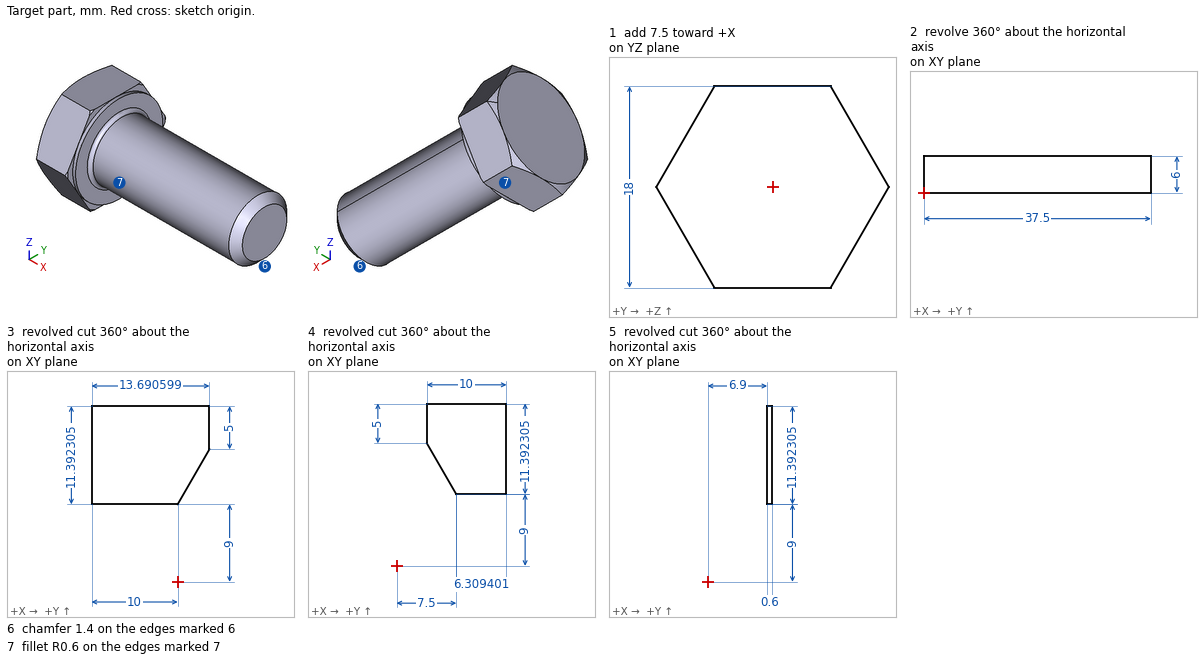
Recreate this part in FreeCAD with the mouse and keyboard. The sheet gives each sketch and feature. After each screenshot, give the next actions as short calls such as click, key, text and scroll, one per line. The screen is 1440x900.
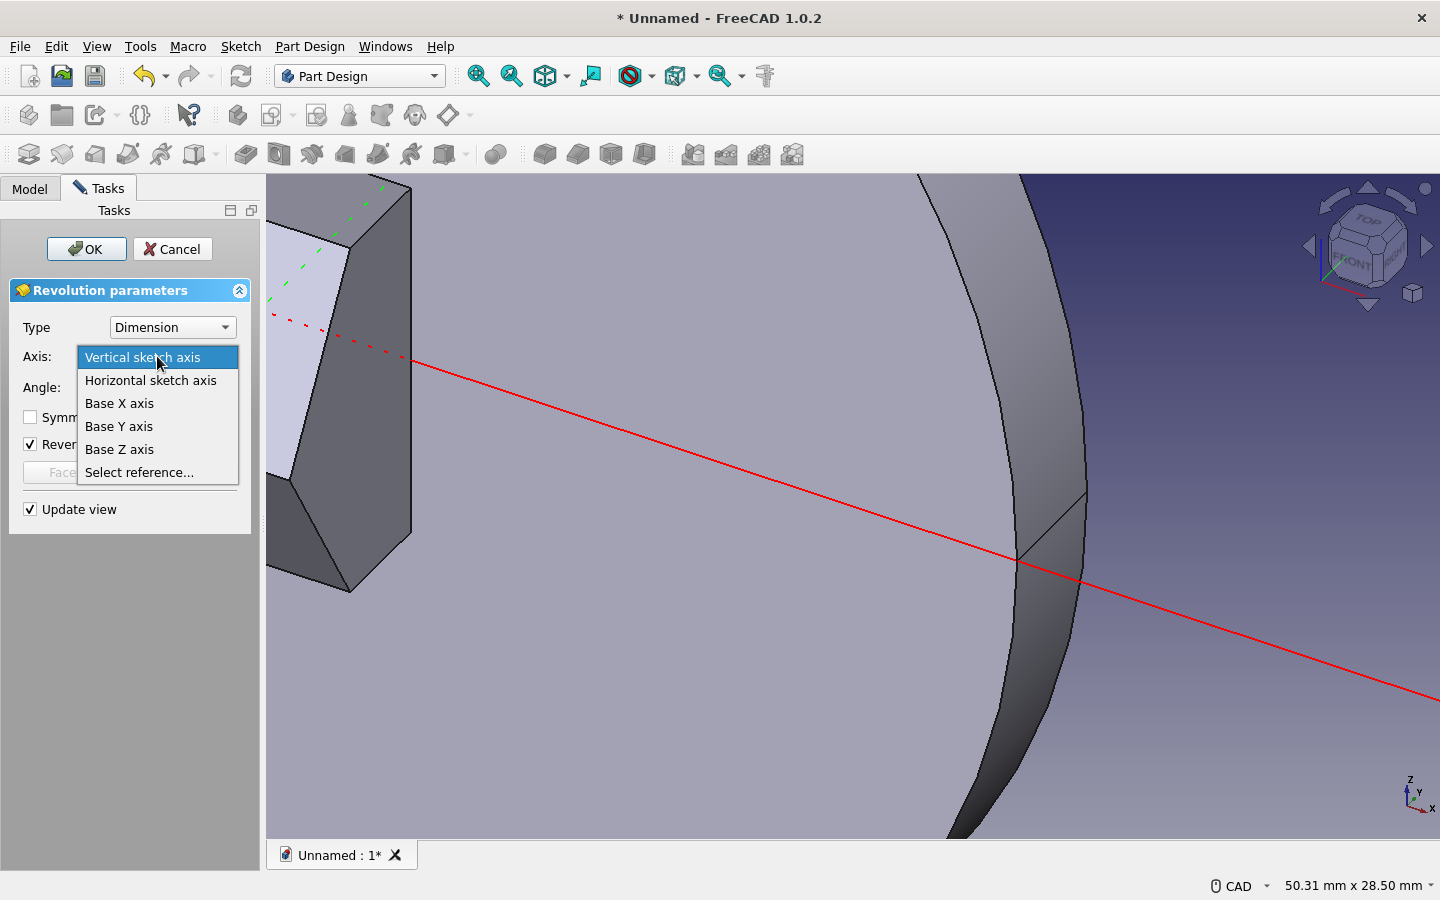
click(156, 380)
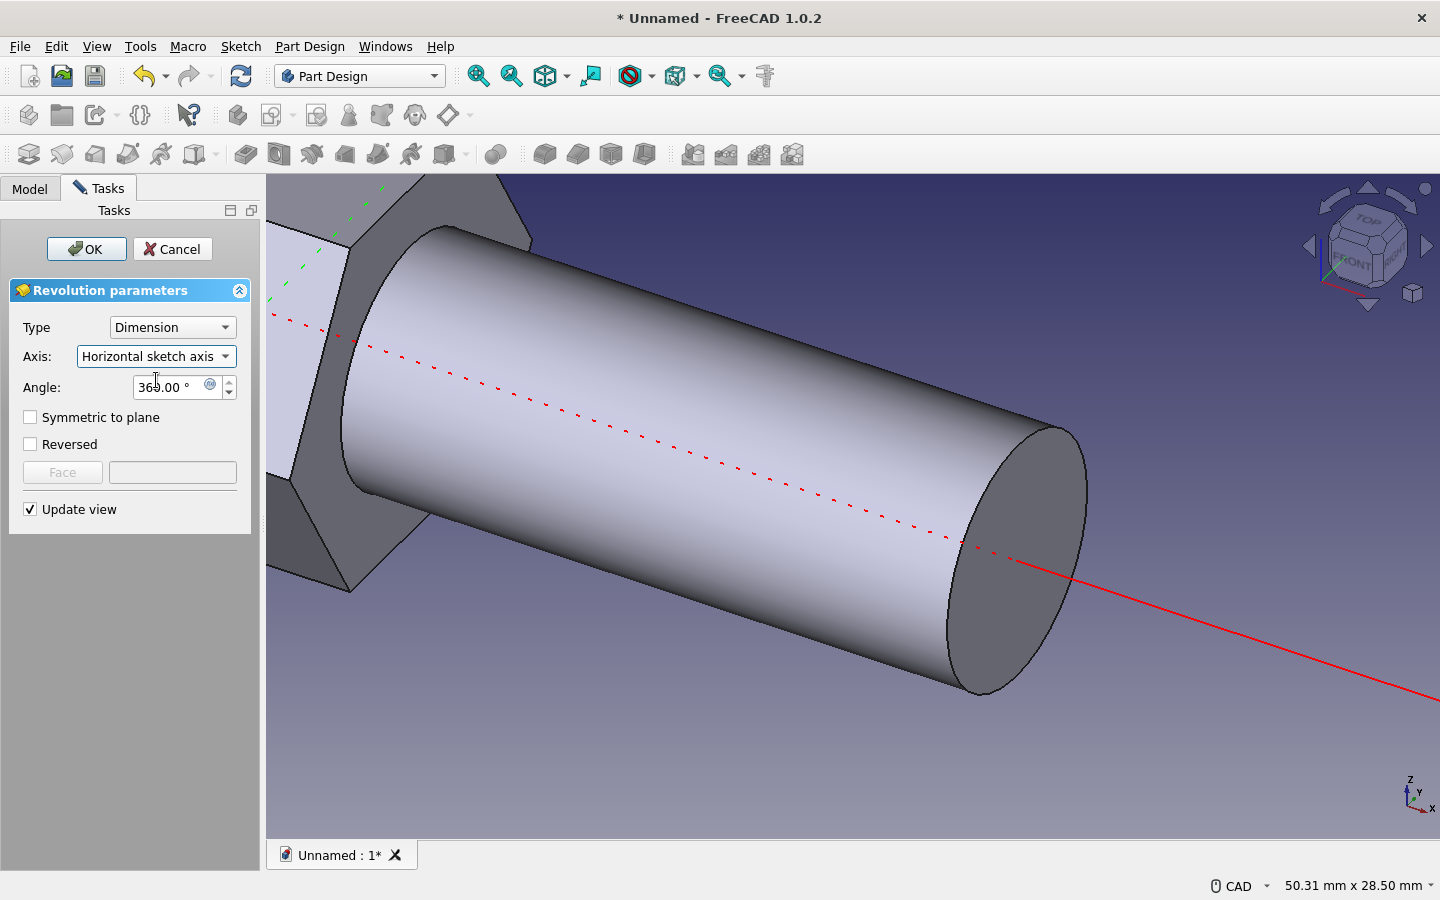
click(87, 249)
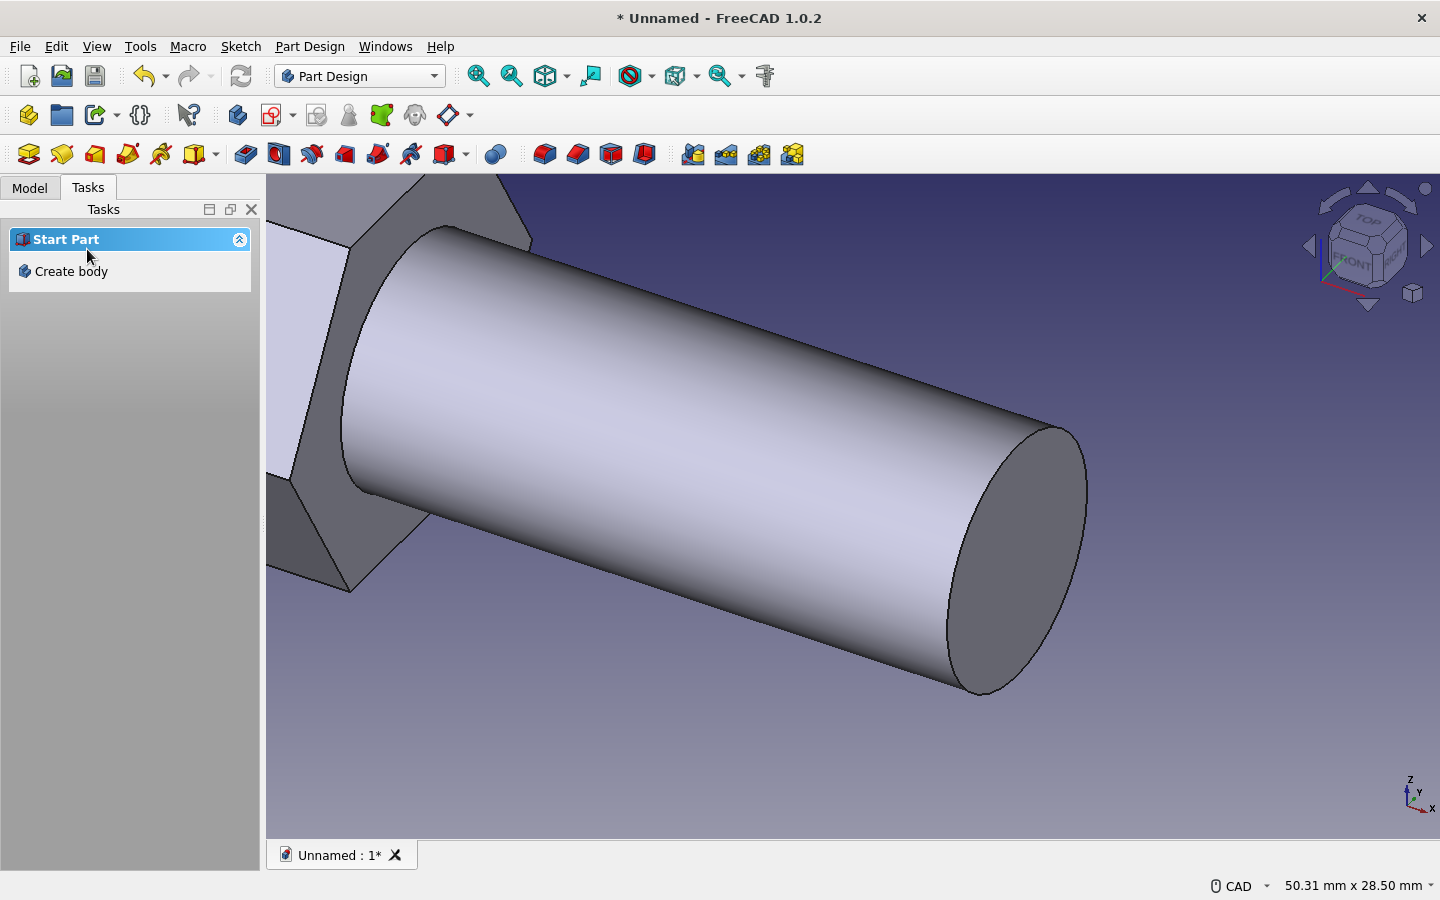
click(479, 76)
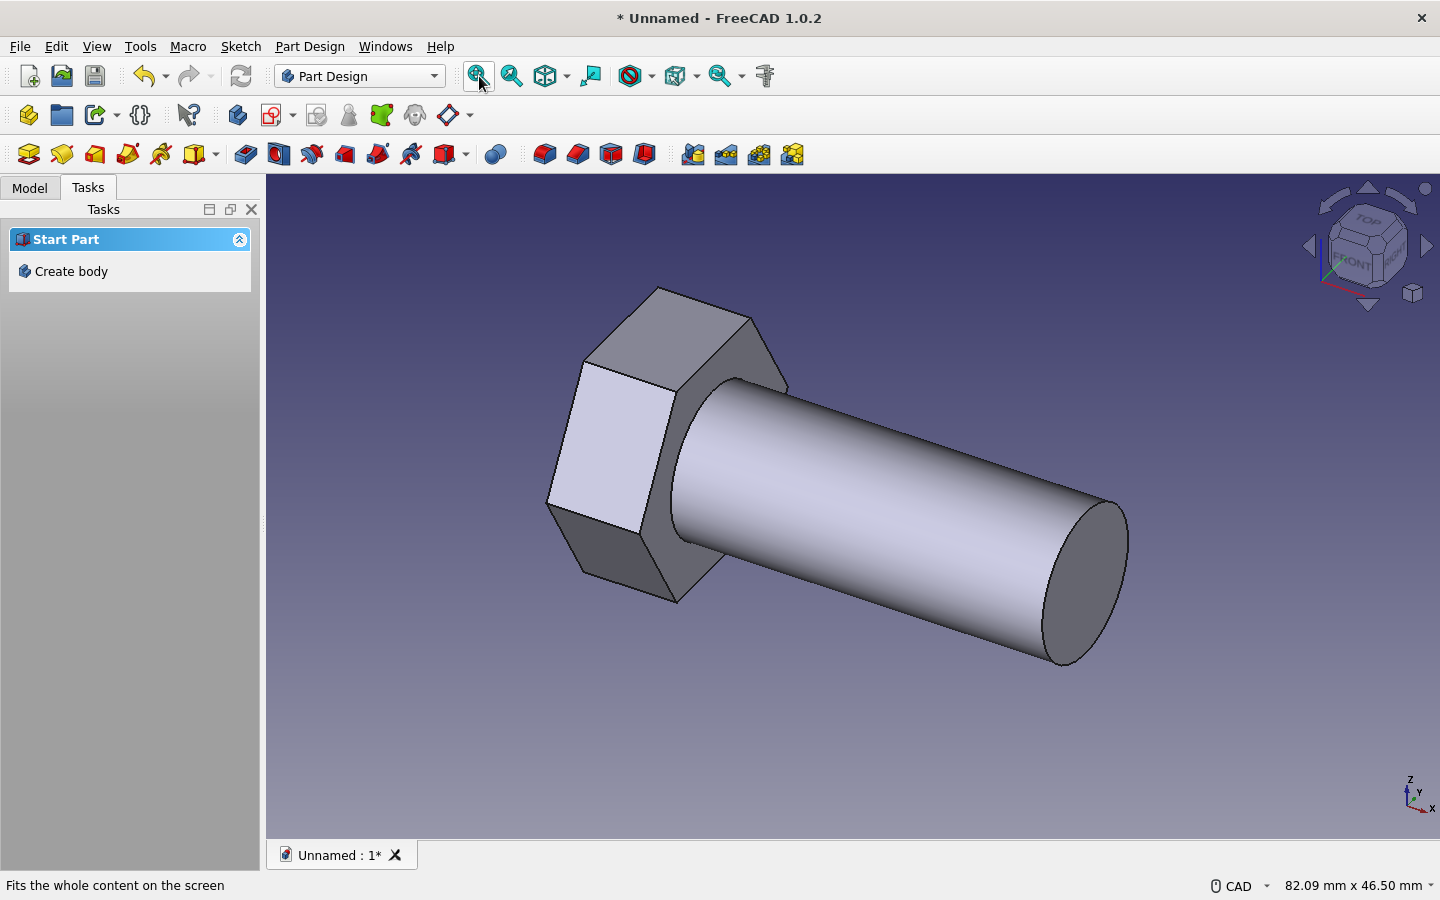
click(270, 116)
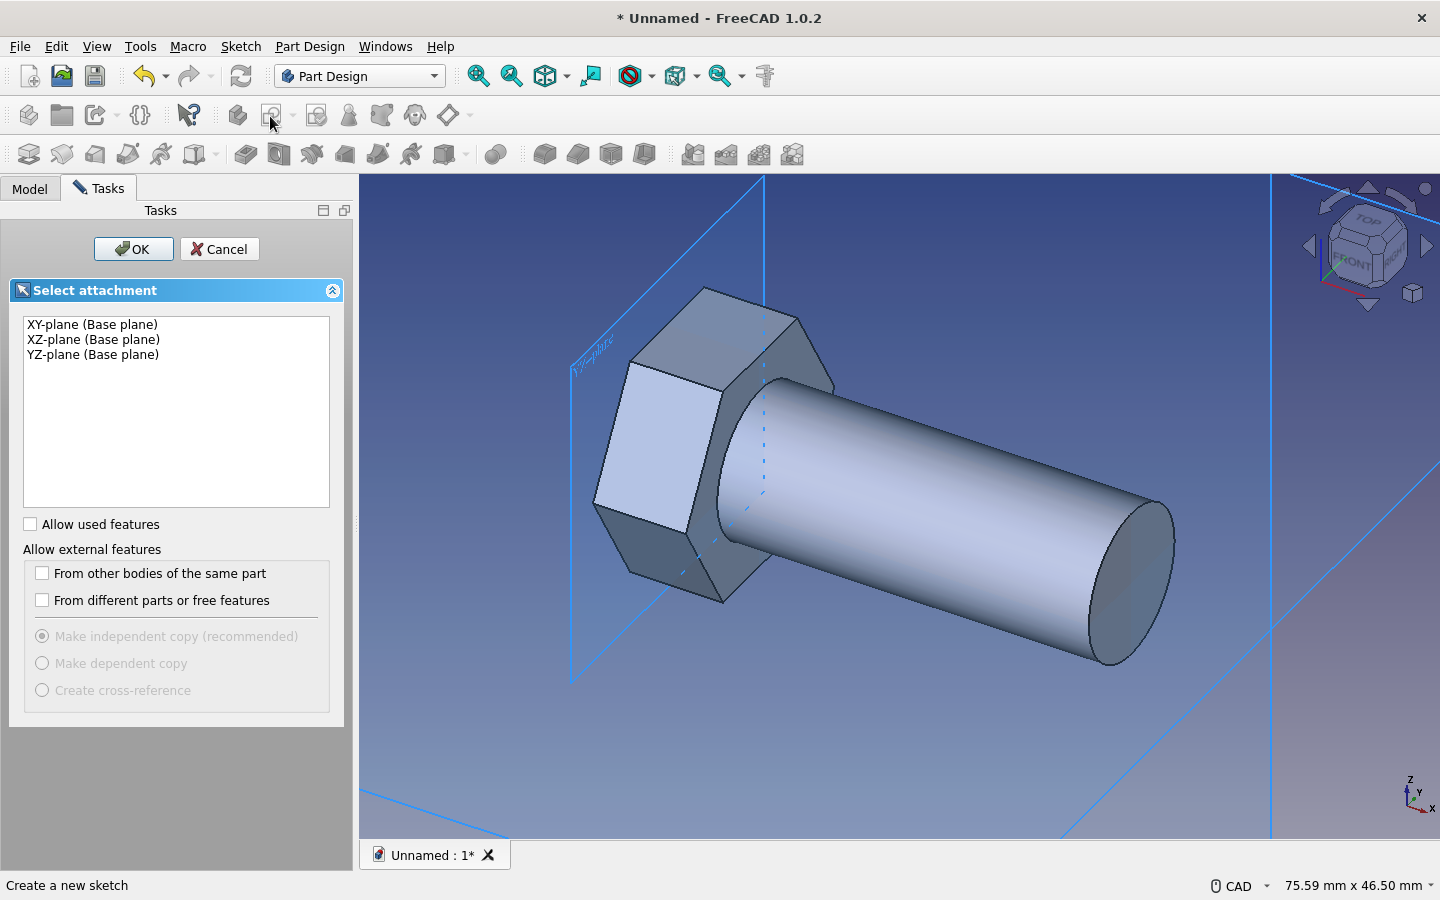
click(84, 324)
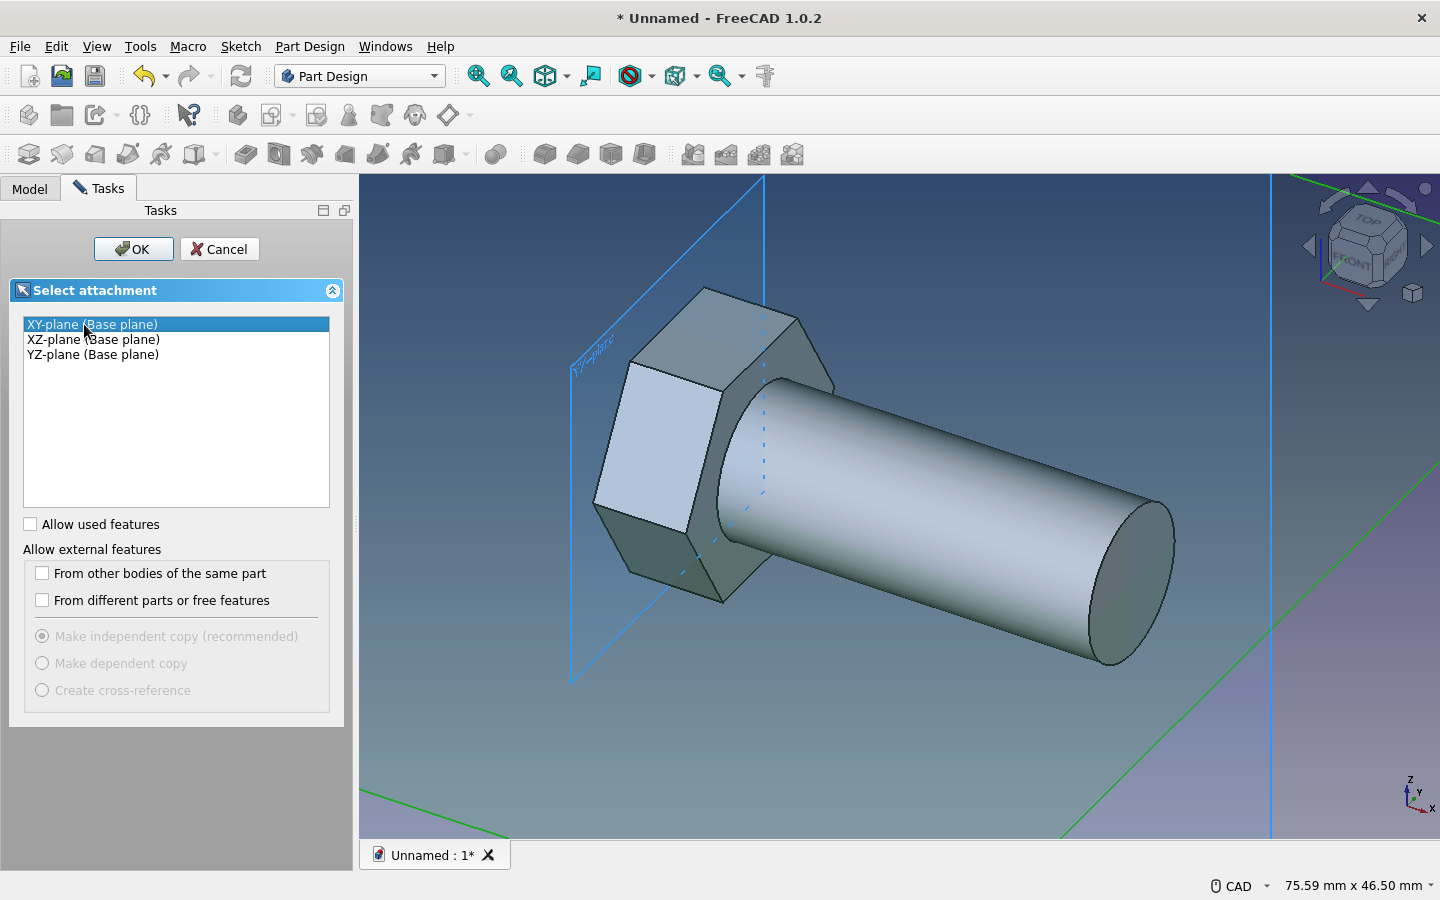
click(134, 249)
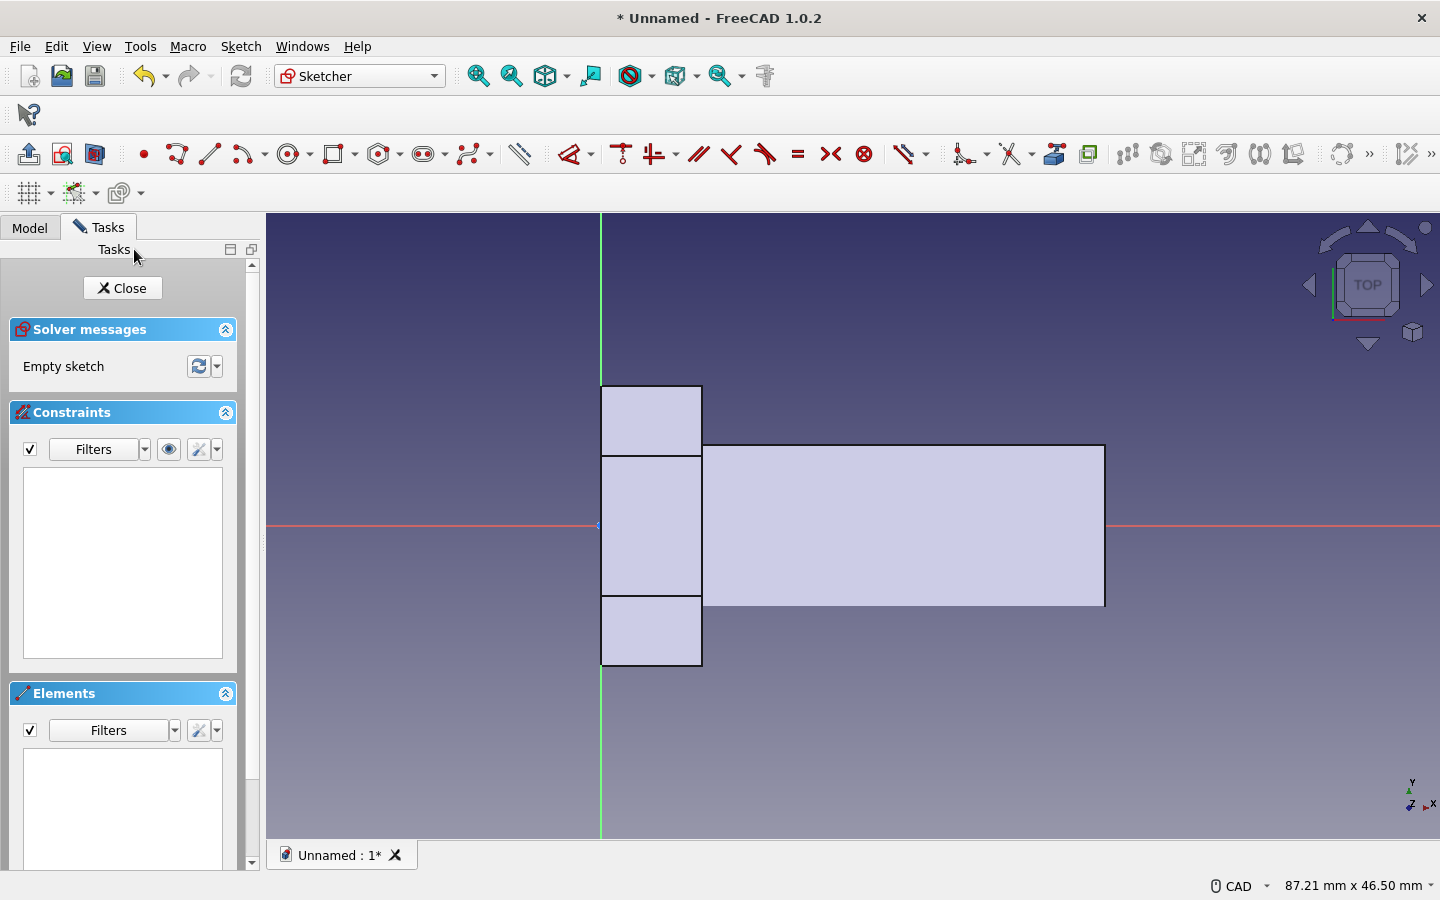
key(q)
key(s)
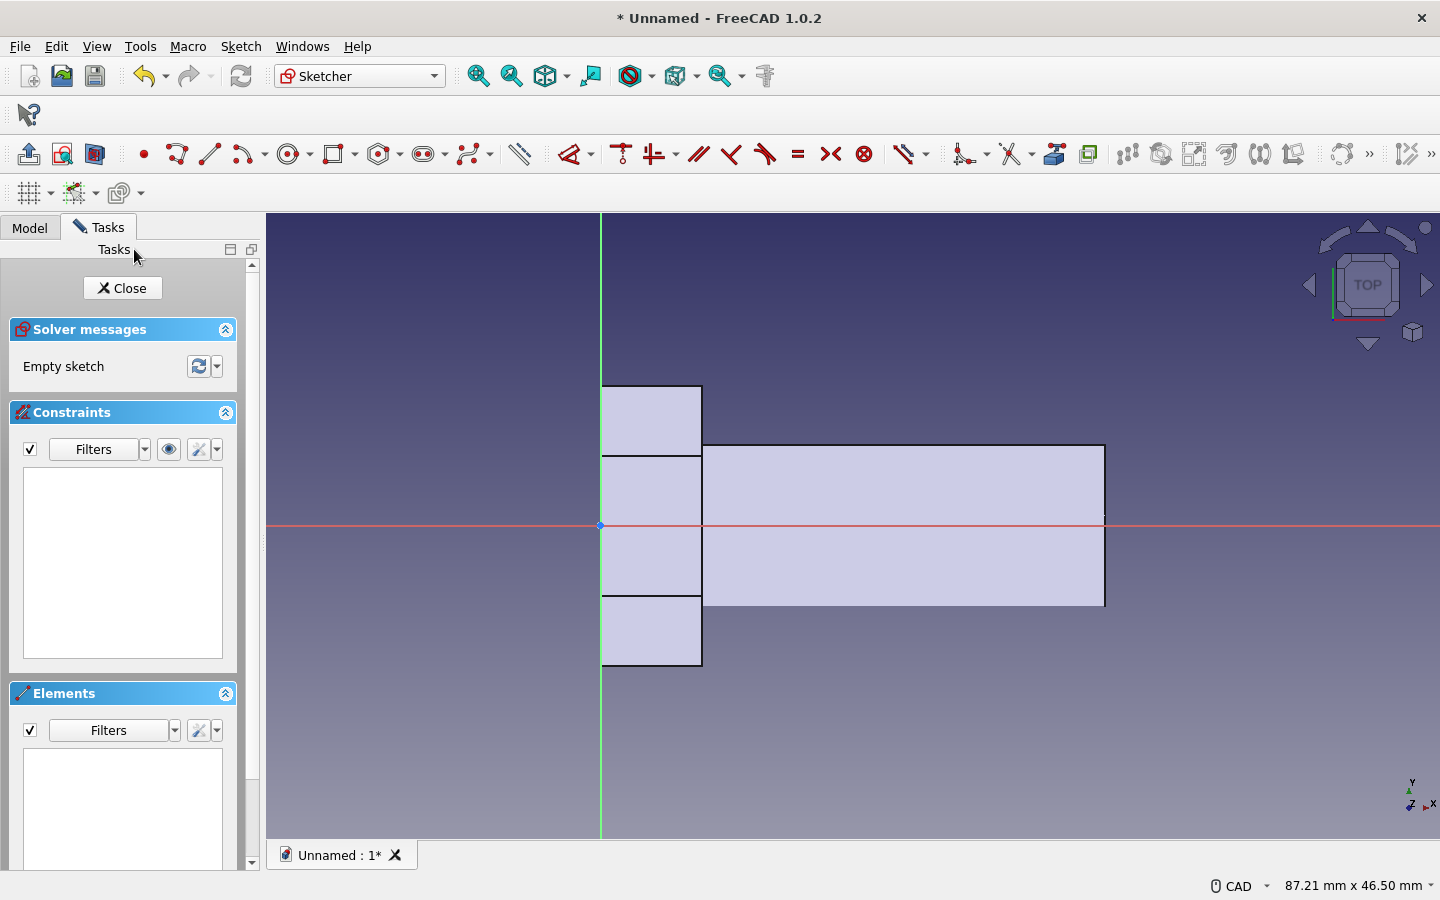
scroll(1275, 811, down, 1)